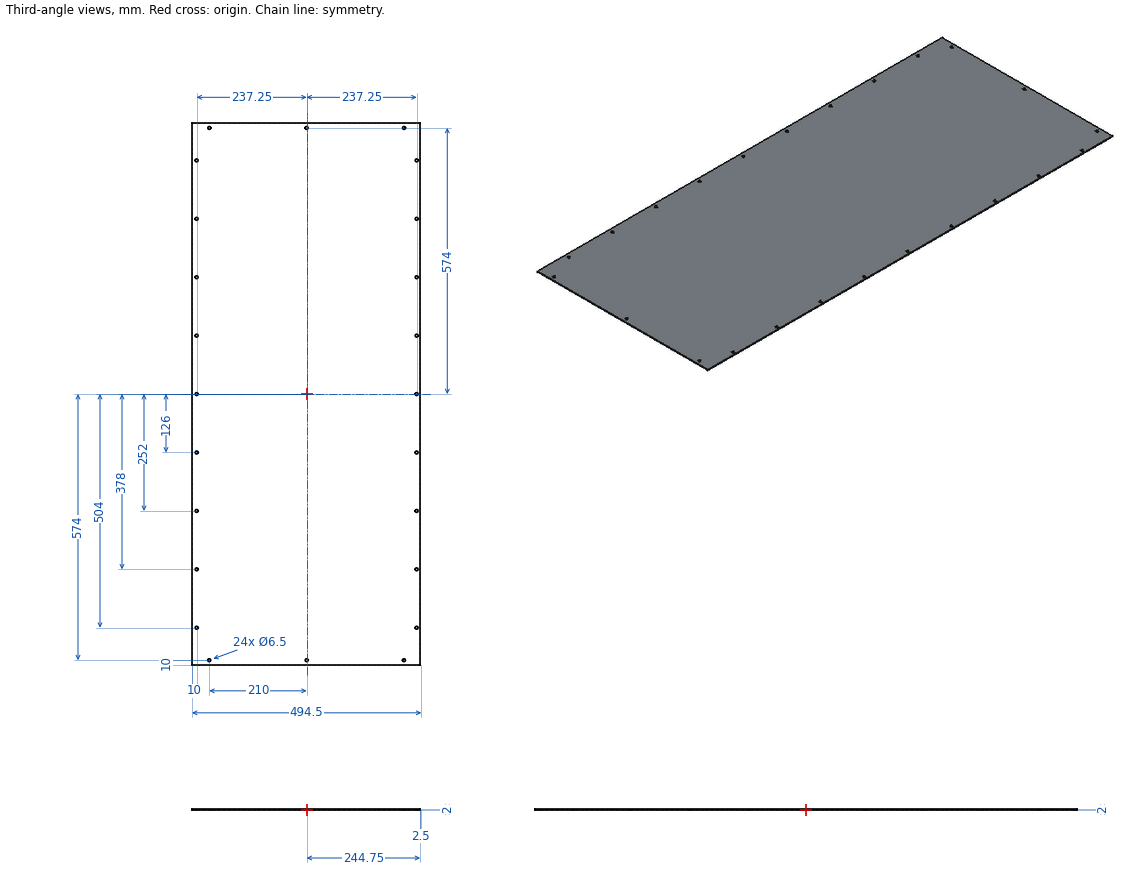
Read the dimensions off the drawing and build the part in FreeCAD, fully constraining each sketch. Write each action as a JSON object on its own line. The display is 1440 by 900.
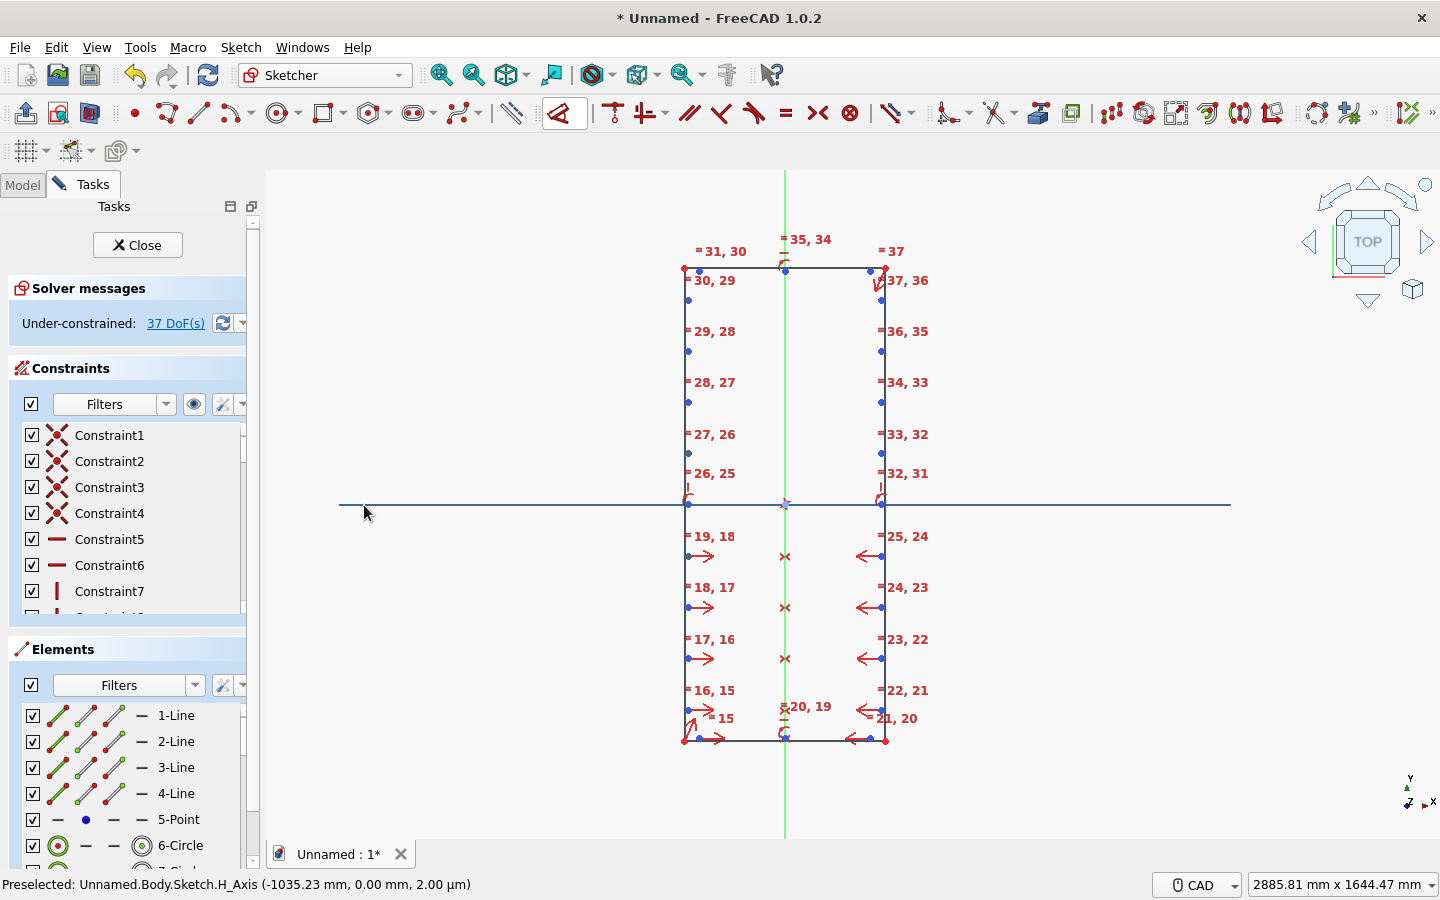
{"action": "key", "text": "s"}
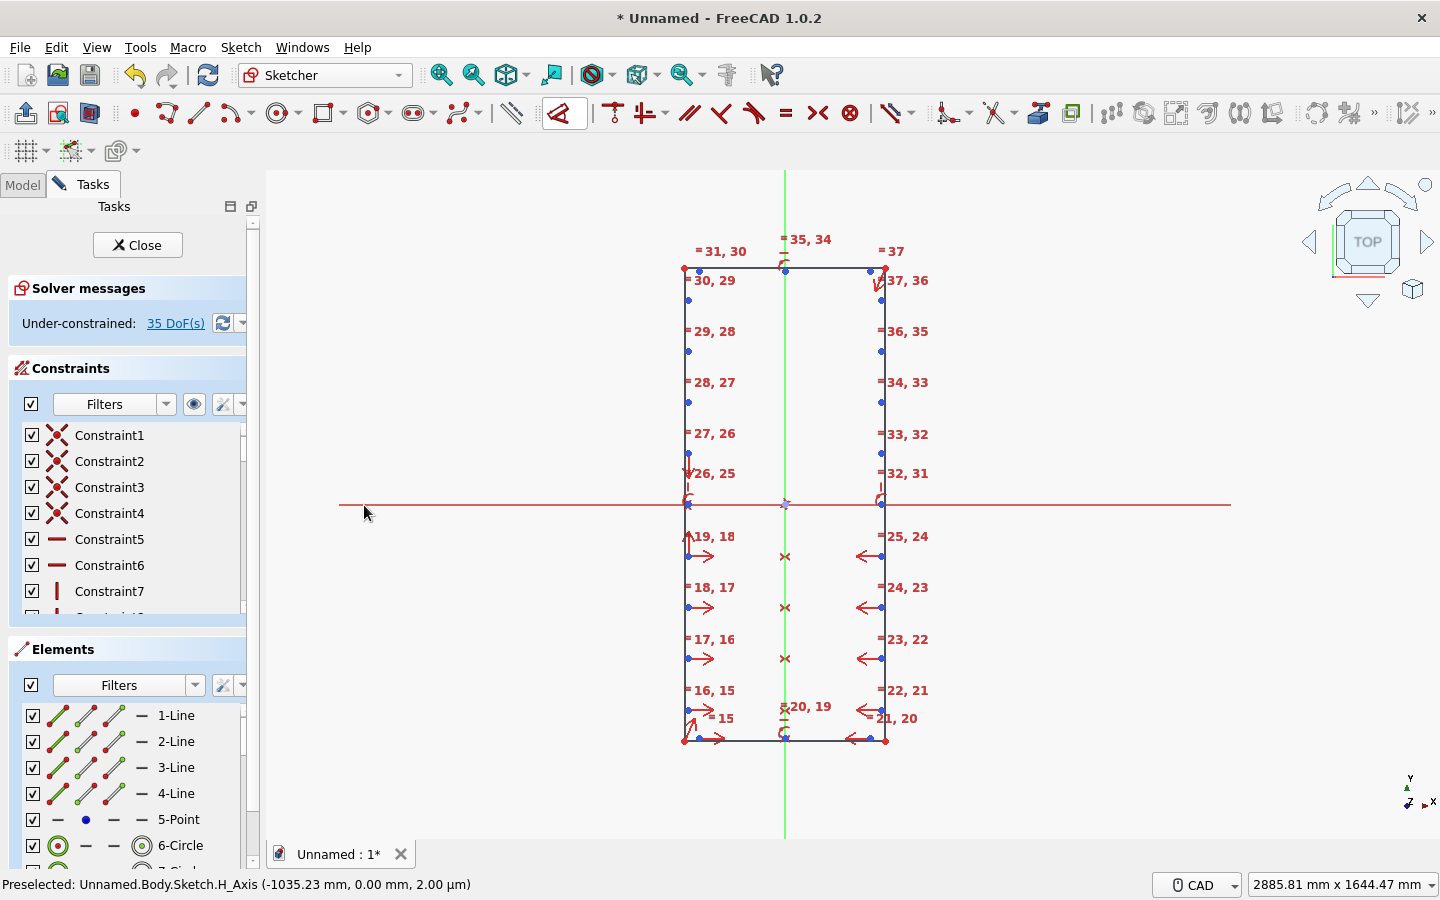
{"action": "left_click", "coordinate": [689, 608]}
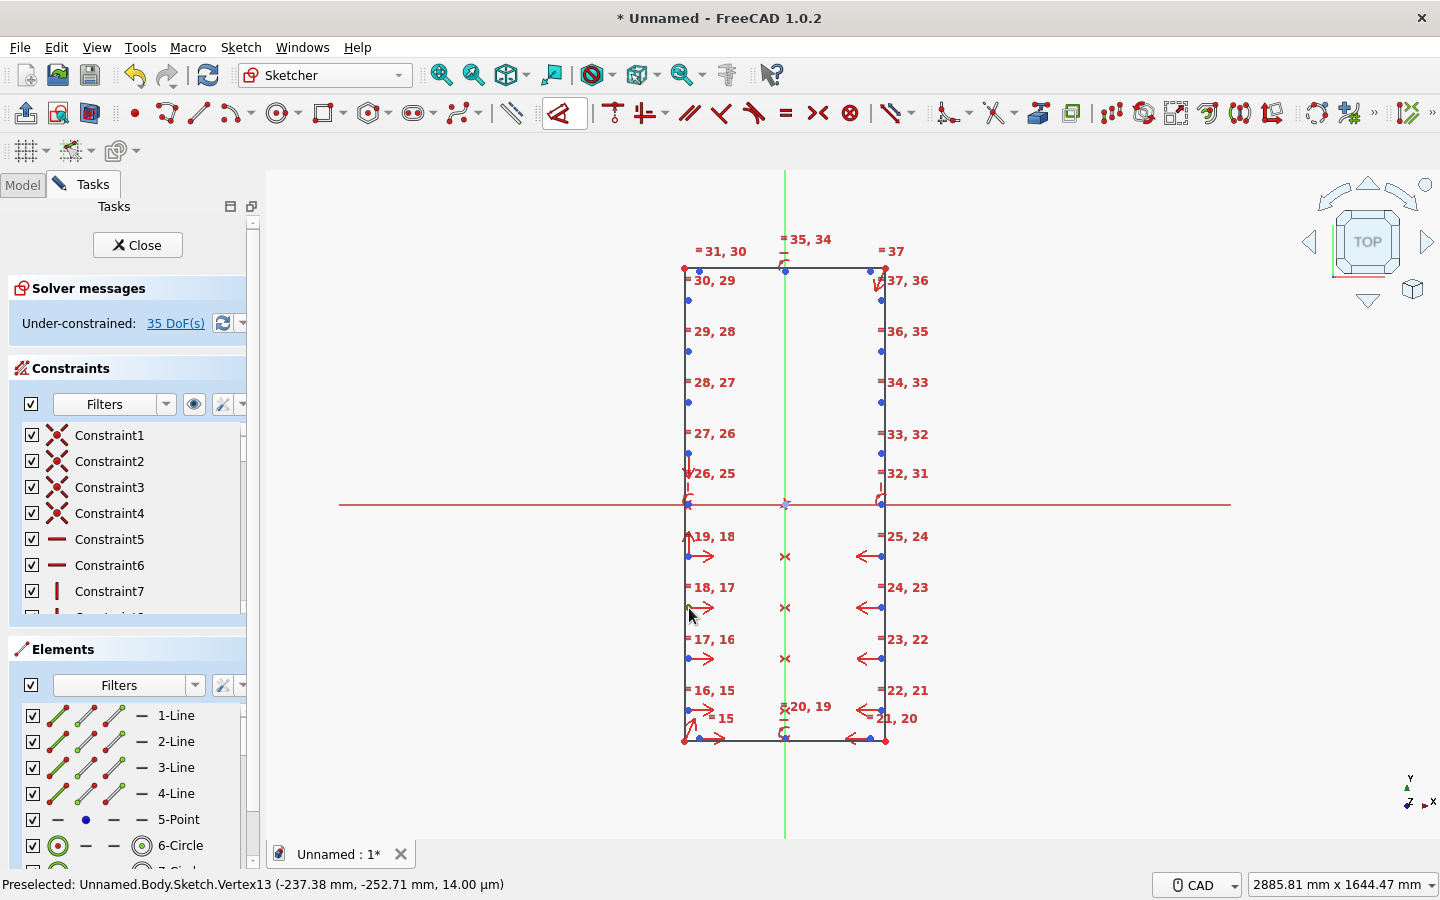
{"action": "left_click", "coordinate": [689, 403]}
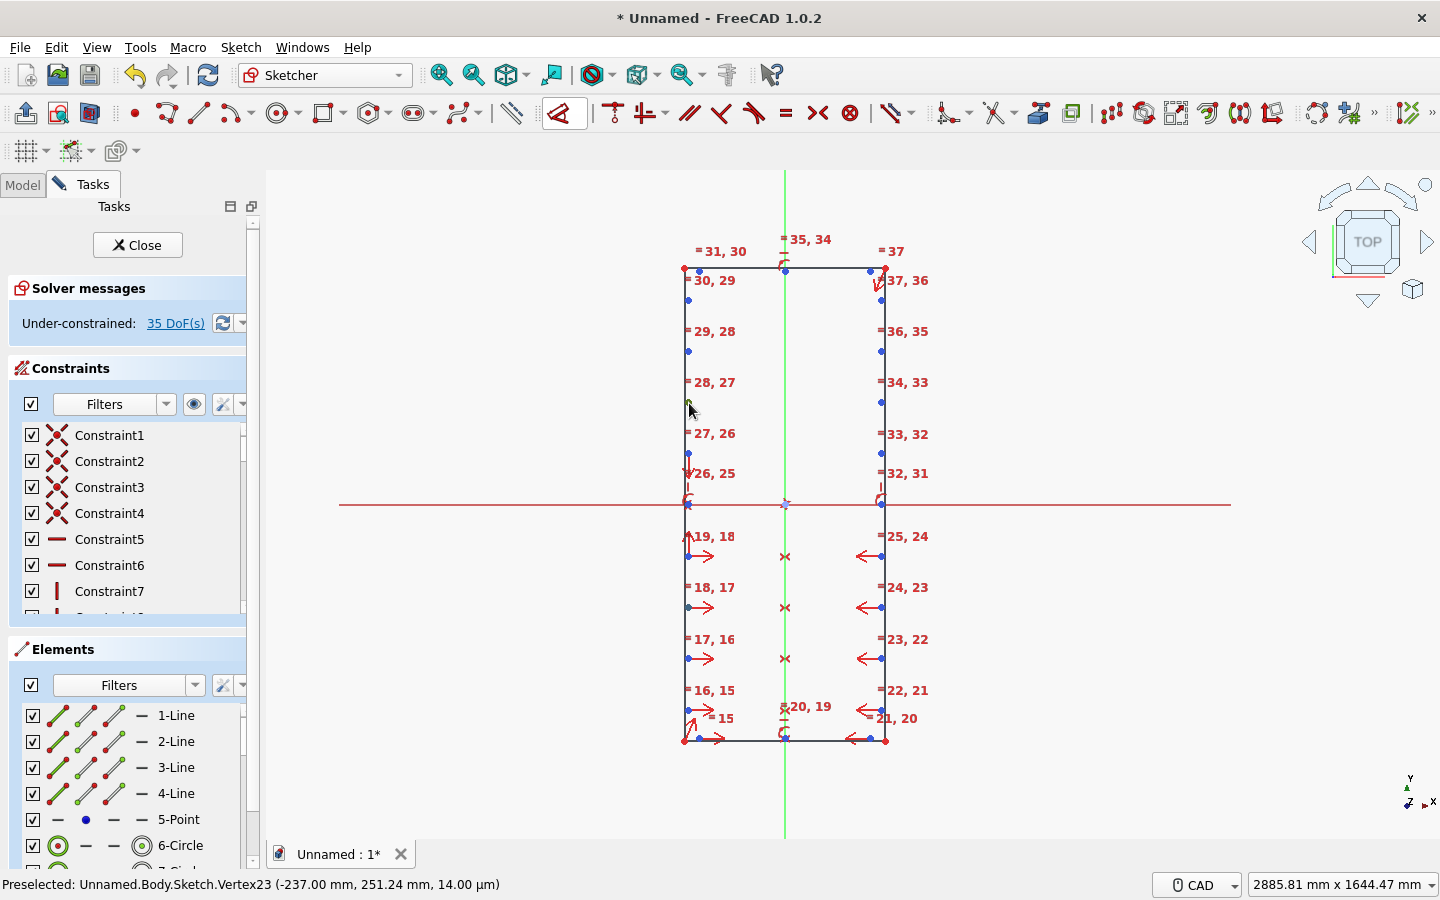
{"action": "left_click", "coordinate": [364, 505]}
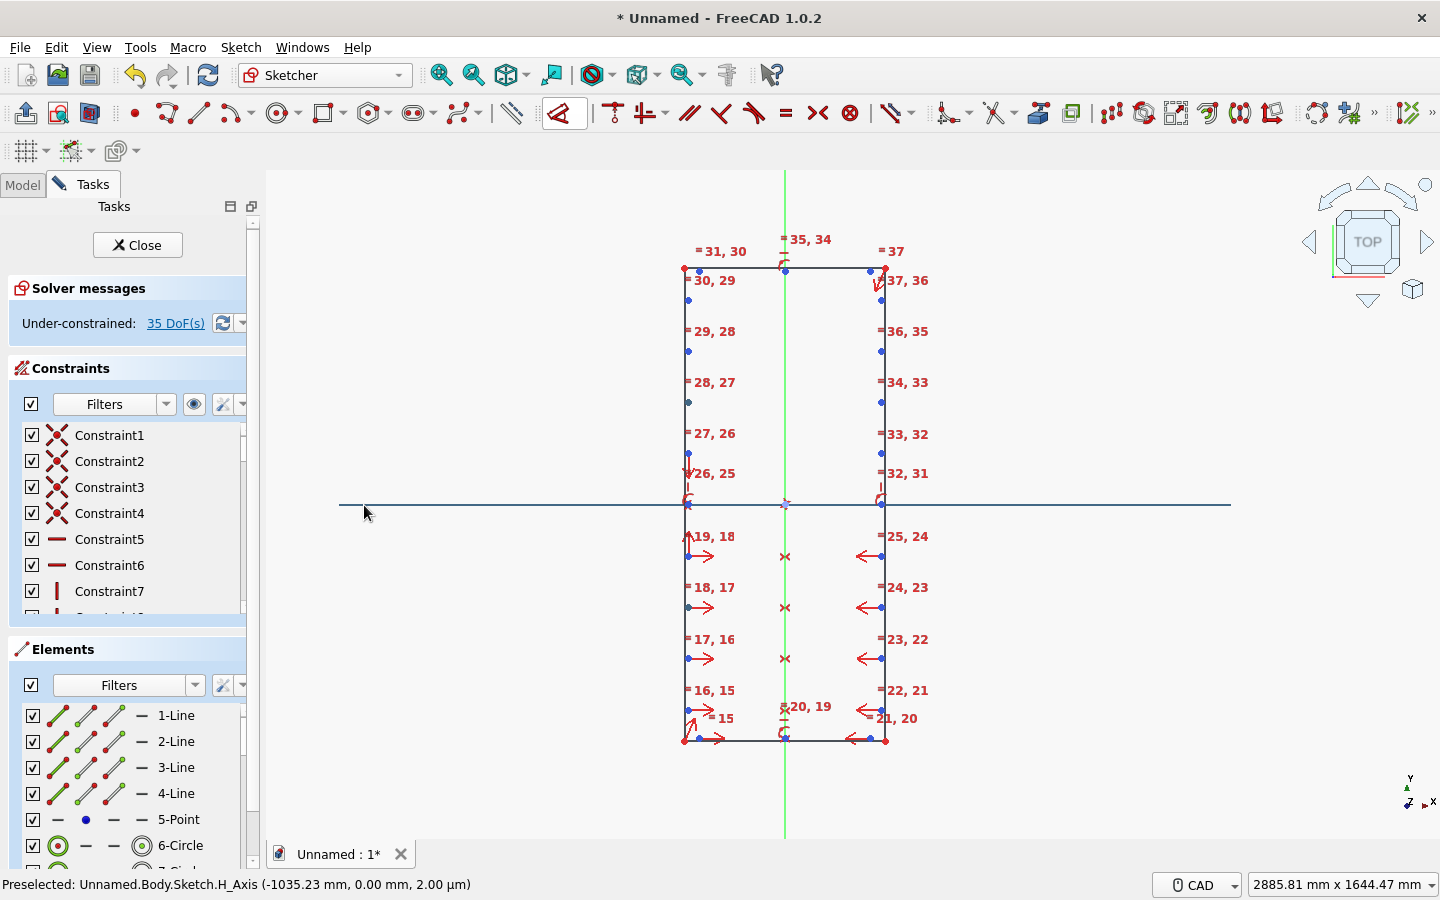
{"action": "key", "text": "s"}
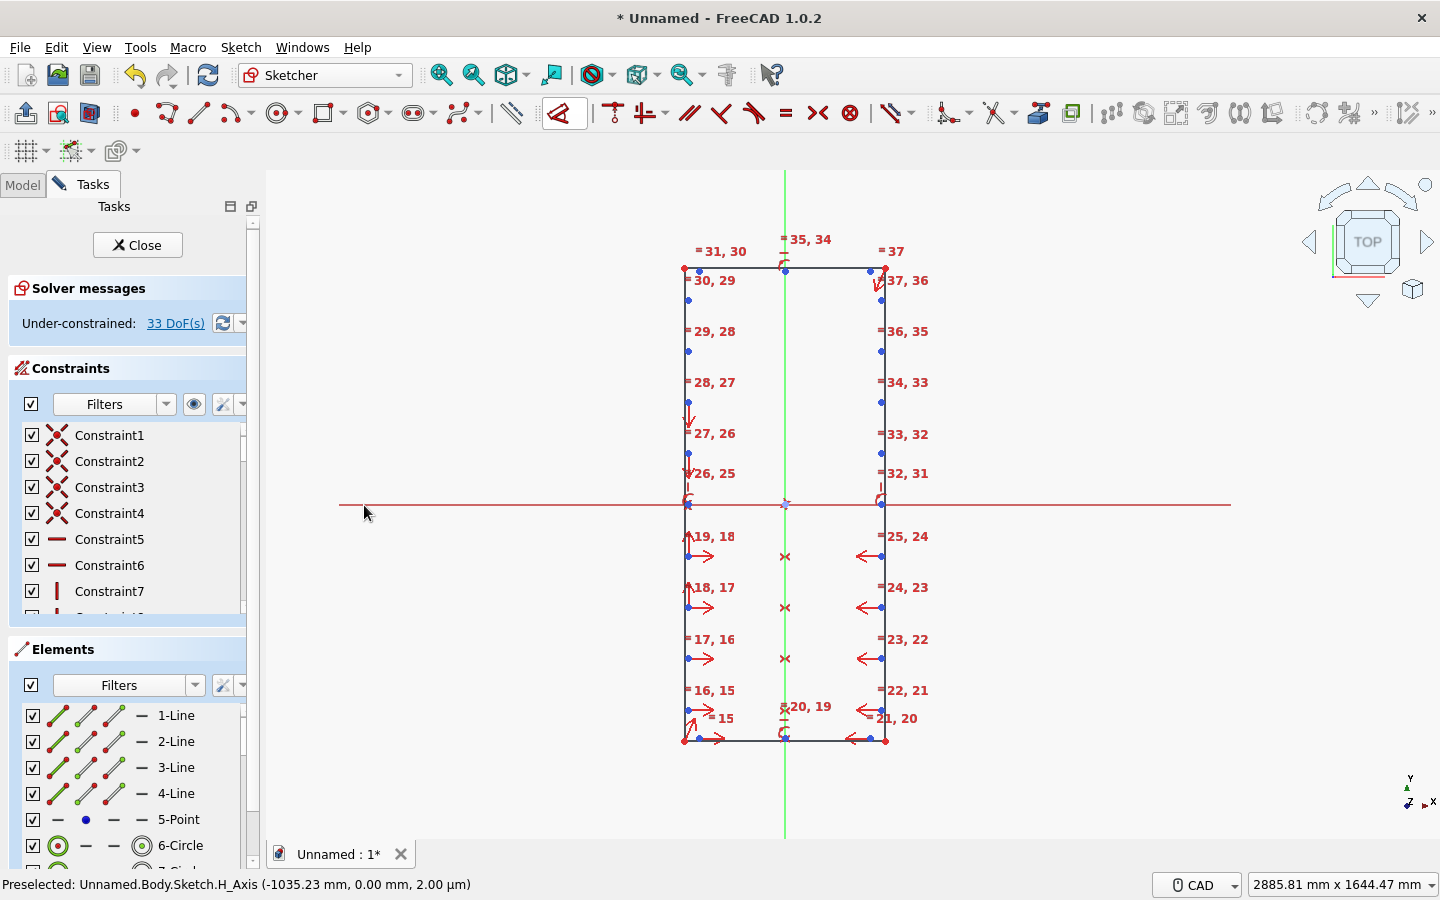
{"action": "left_click", "coordinate": [689, 659]}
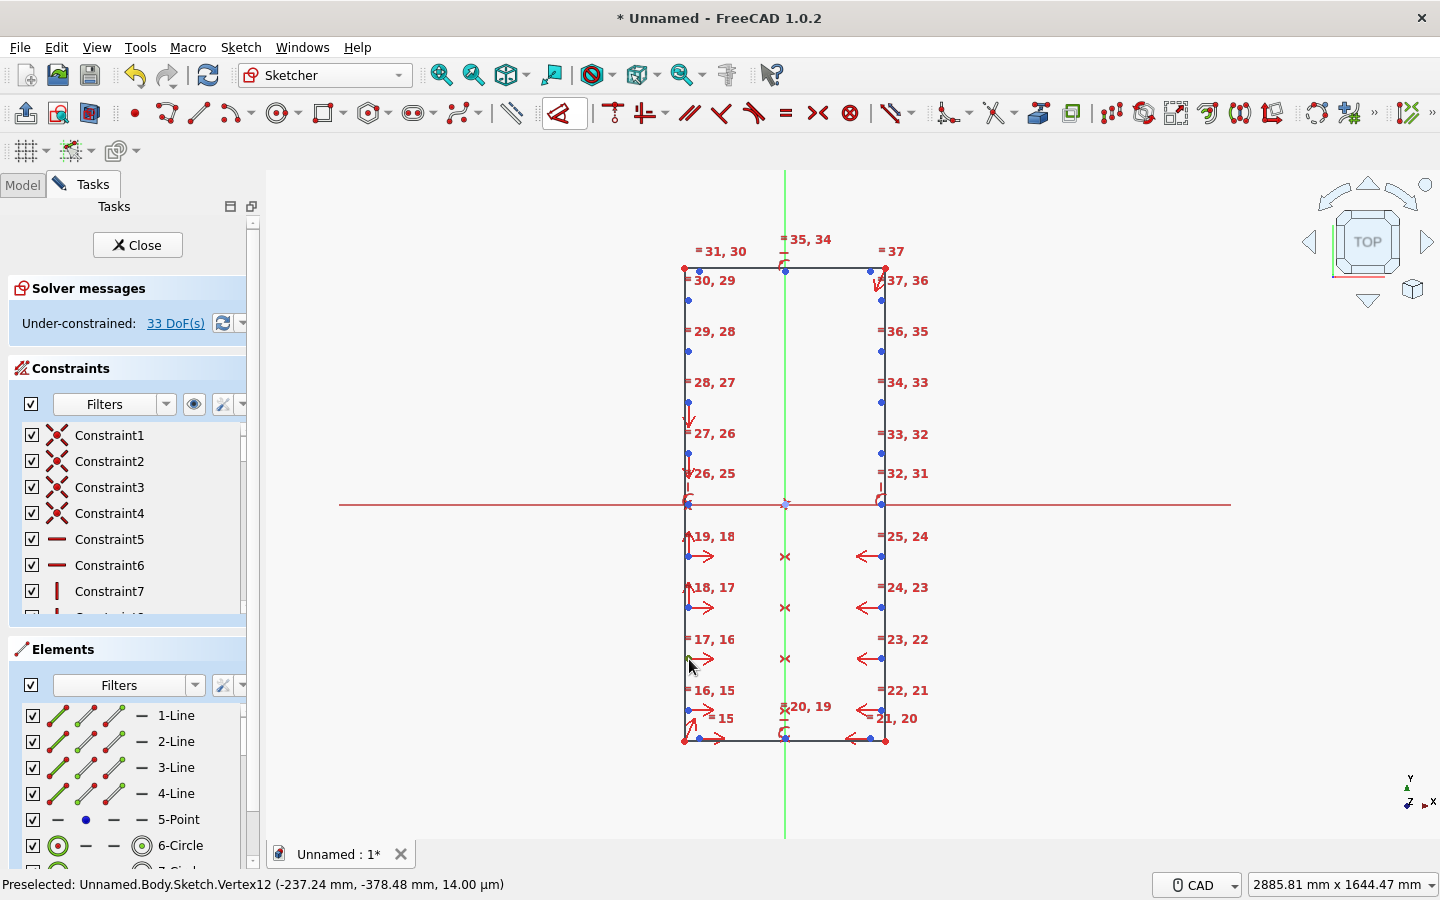
{"action": "left_click", "coordinate": [689, 351]}